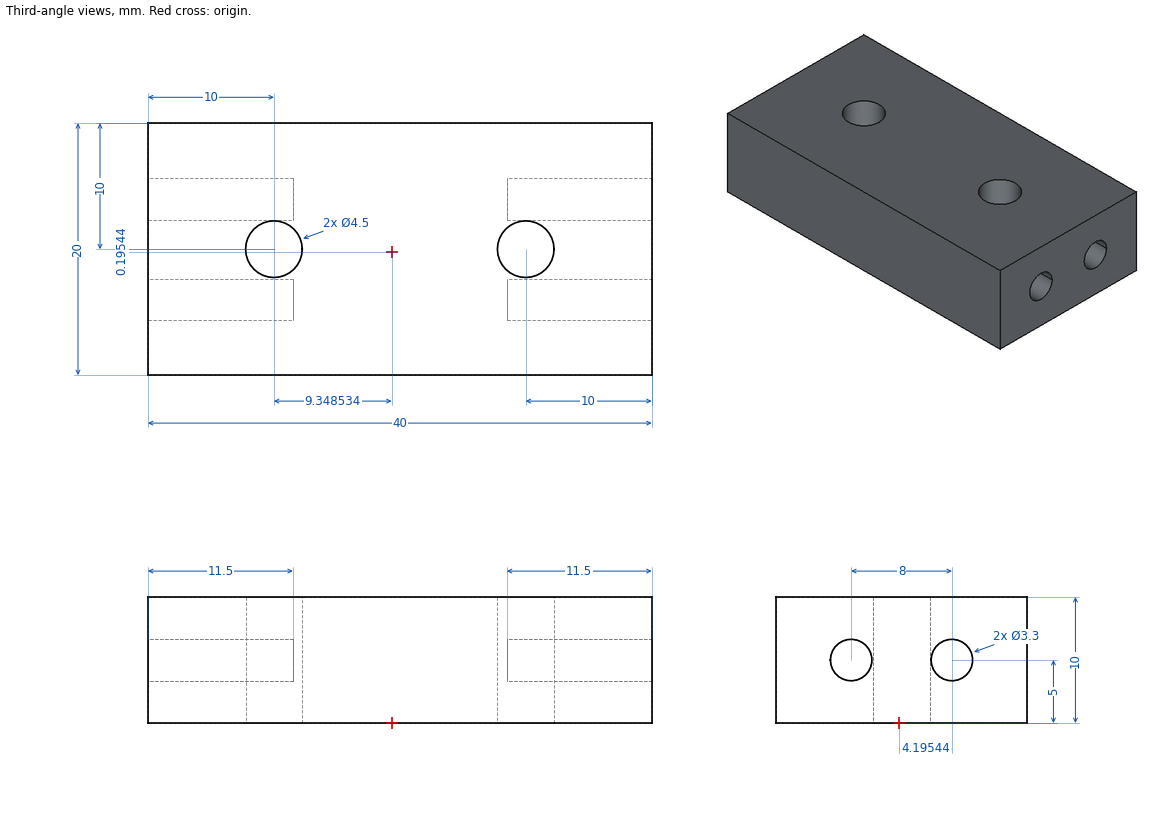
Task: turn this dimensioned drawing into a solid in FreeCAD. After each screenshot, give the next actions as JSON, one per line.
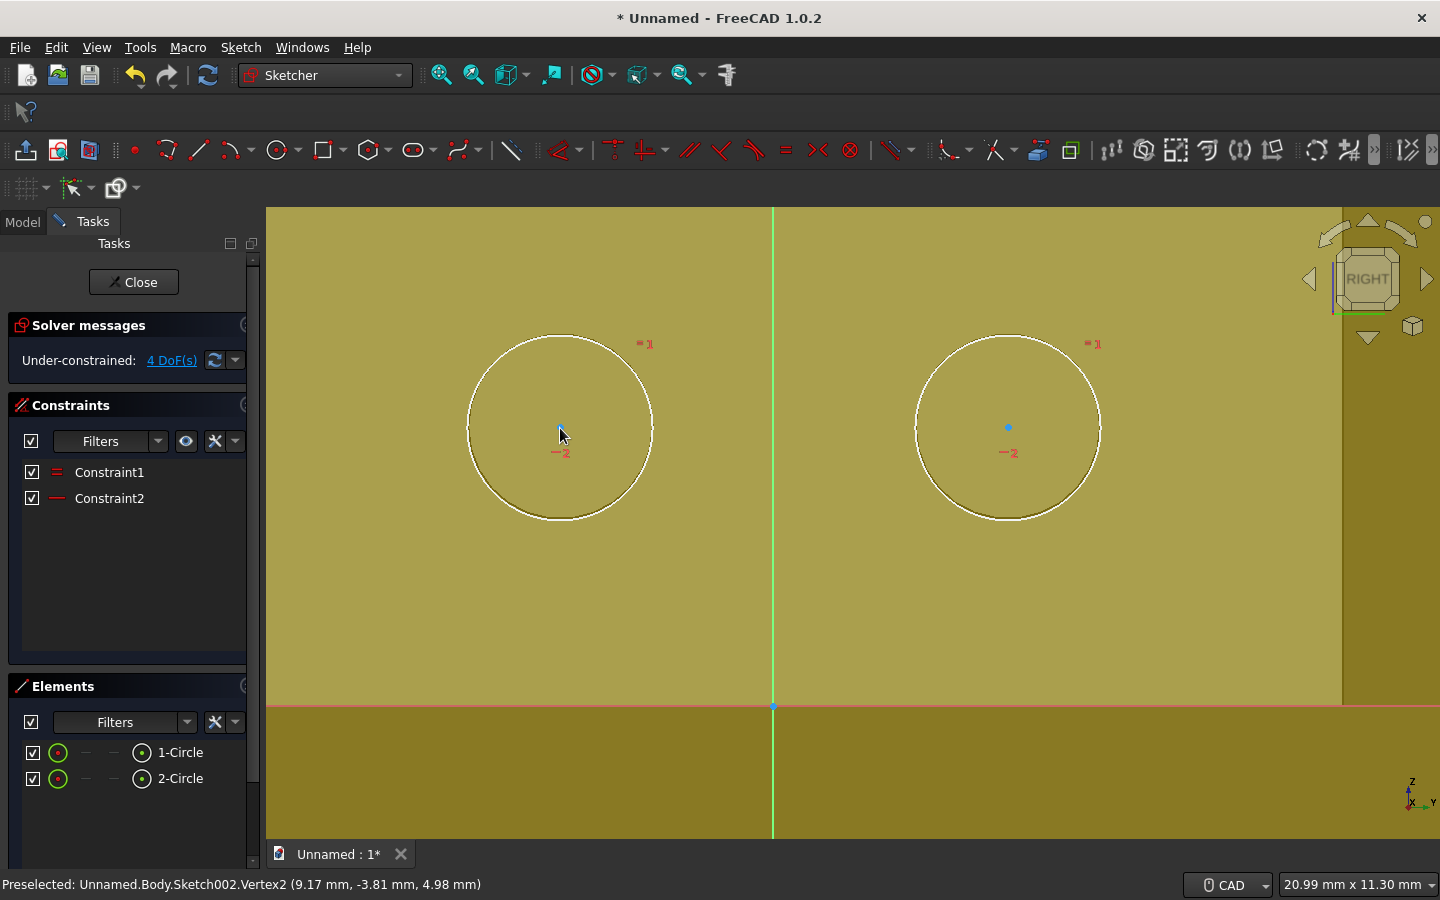
{"action": "key", "text": "d"}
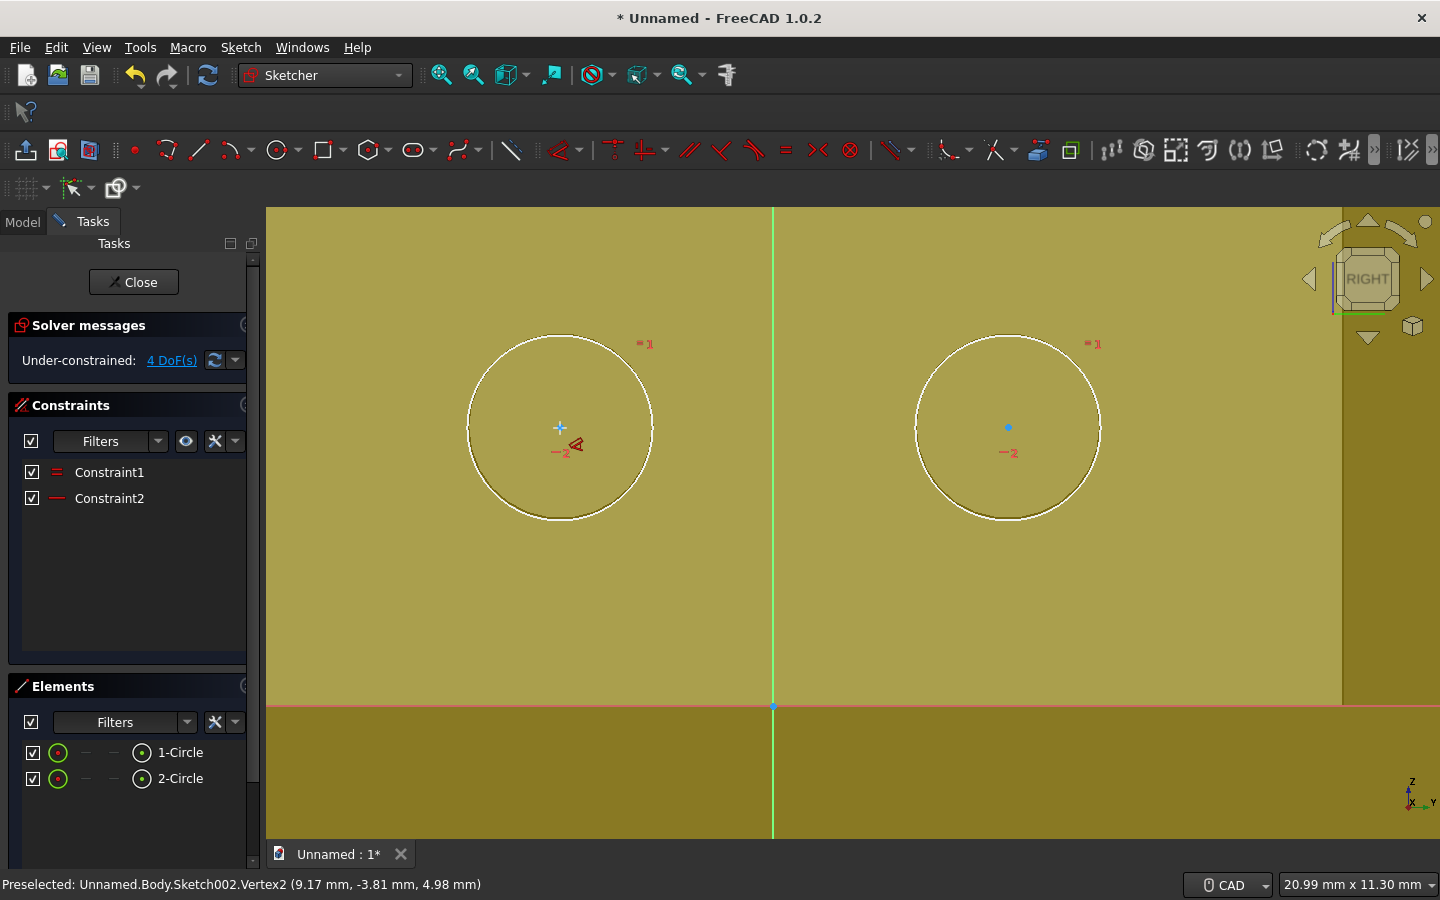
{"action": "left_click", "coordinate": [1073, 362]}
{"action": "left_click", "coordinate": [1095, 339]}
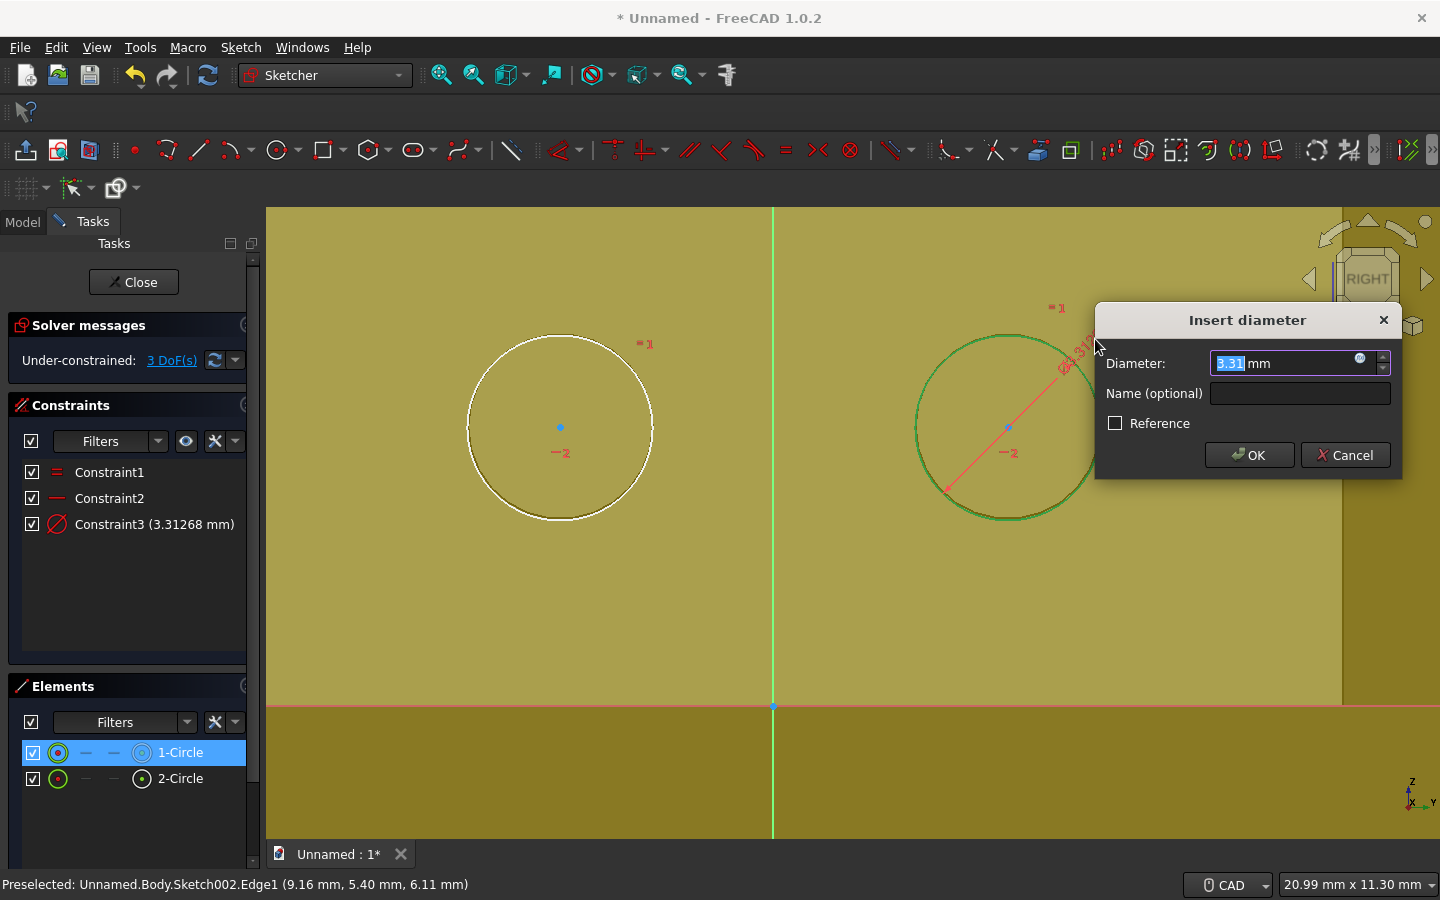
{"action": "type", "text": "3.3"}
{"action": "key", "text": "Return"}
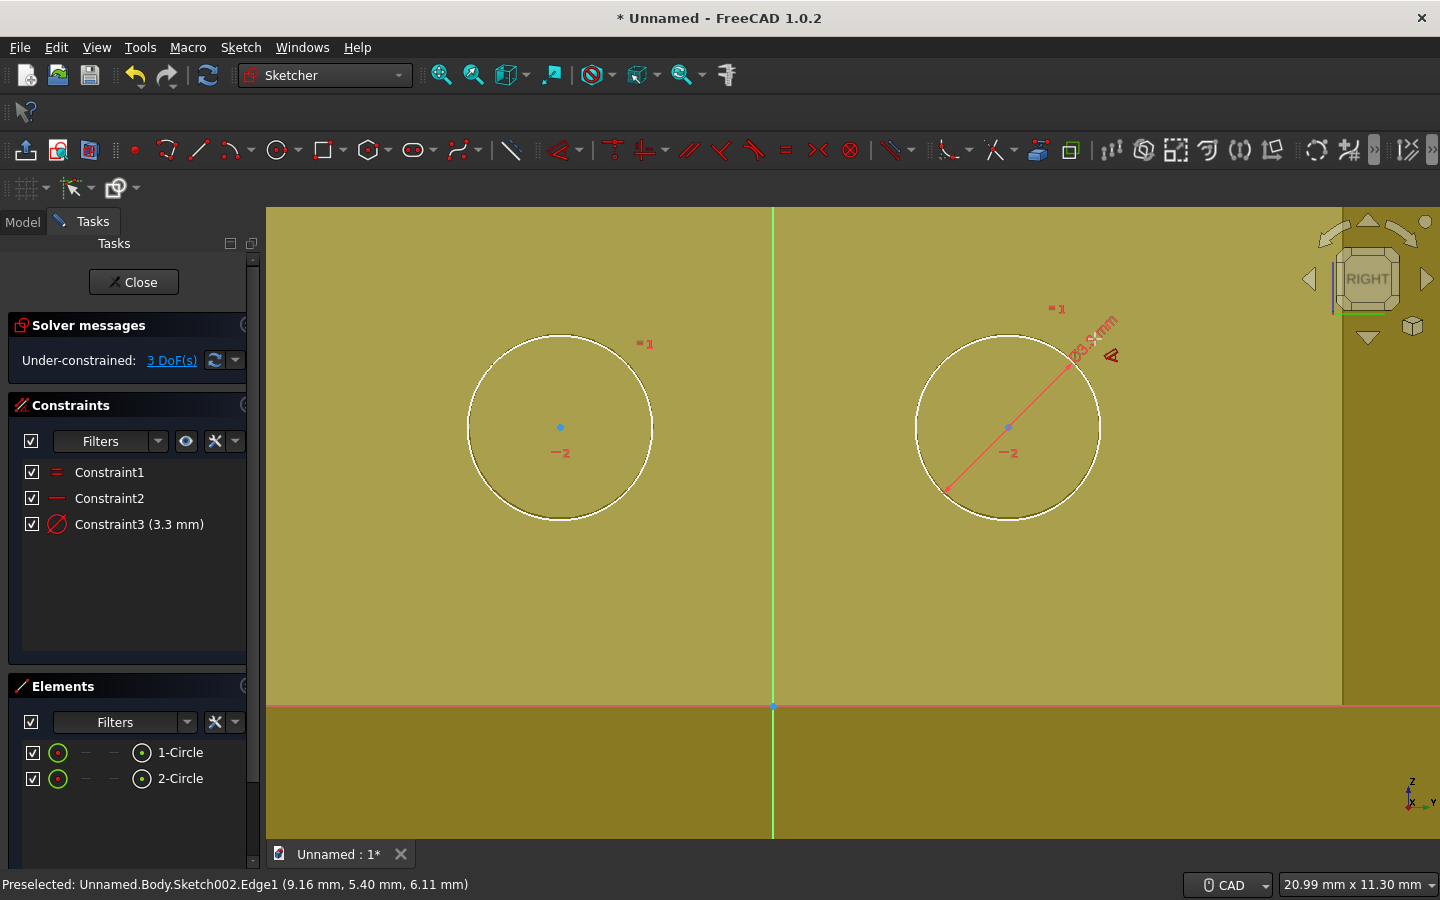
{"action": "left_click", "coordinate": [1008, 428]}
{"action": "left_click", "coordinate": [1042, 567]}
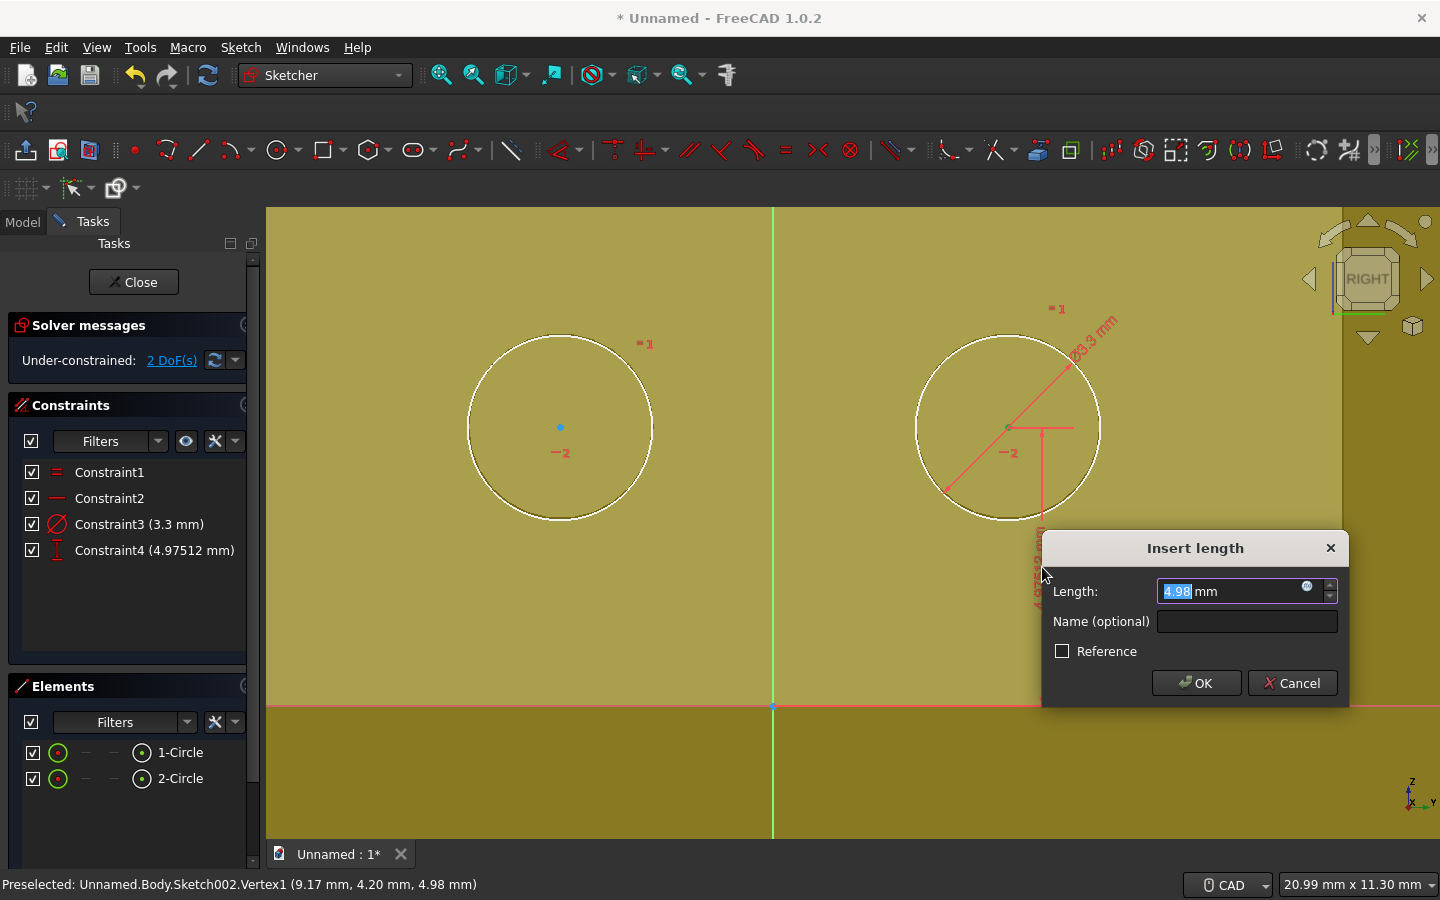
{"action": "type", "text": "5"}
{"action": "key", "text": "Return"}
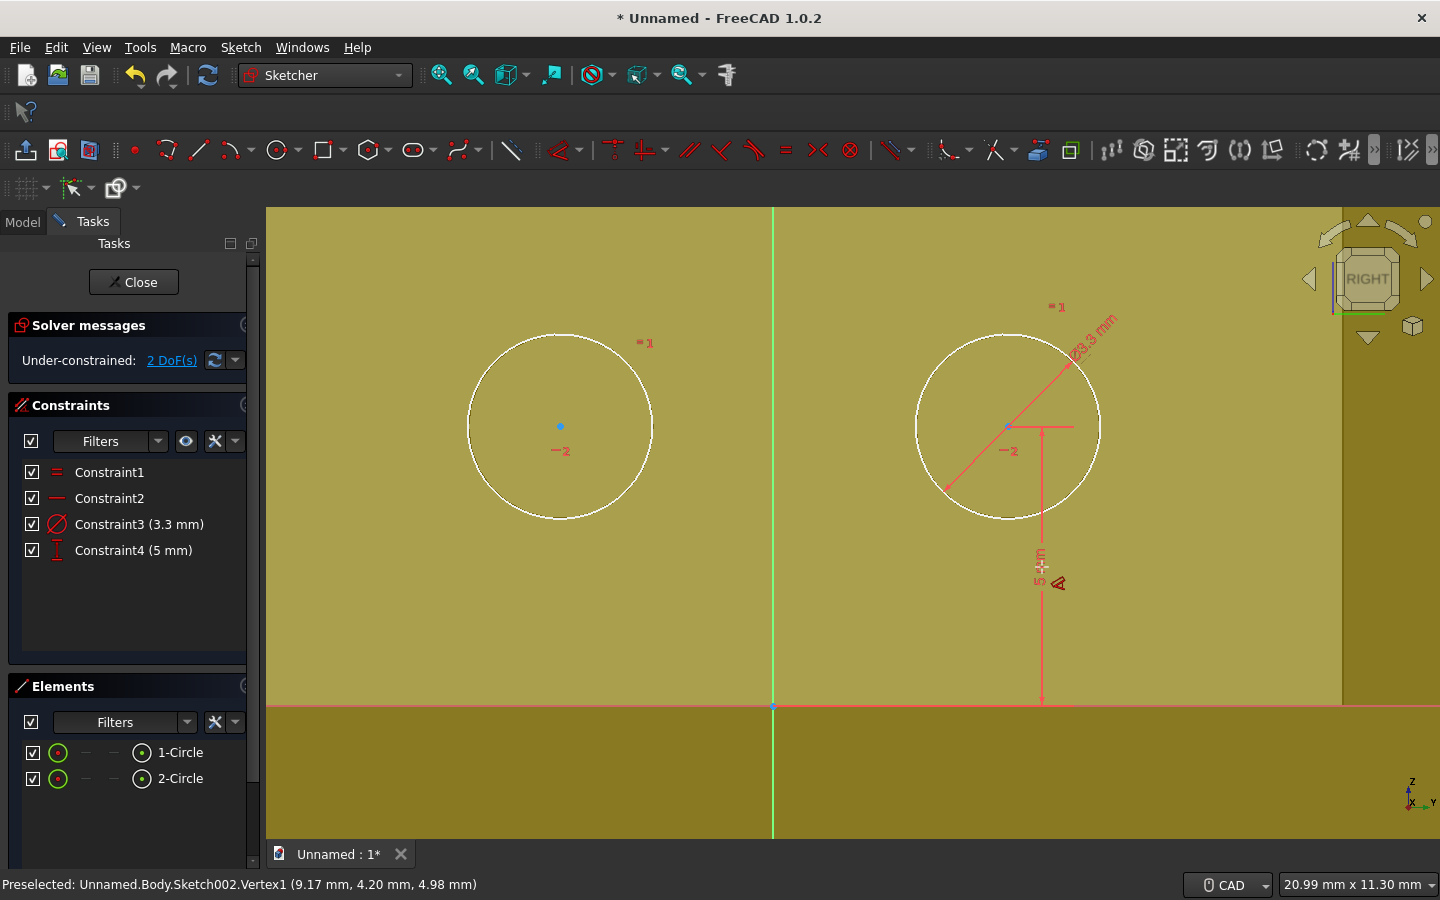
{"action": "left_click", "coordinate": [1008, 427]}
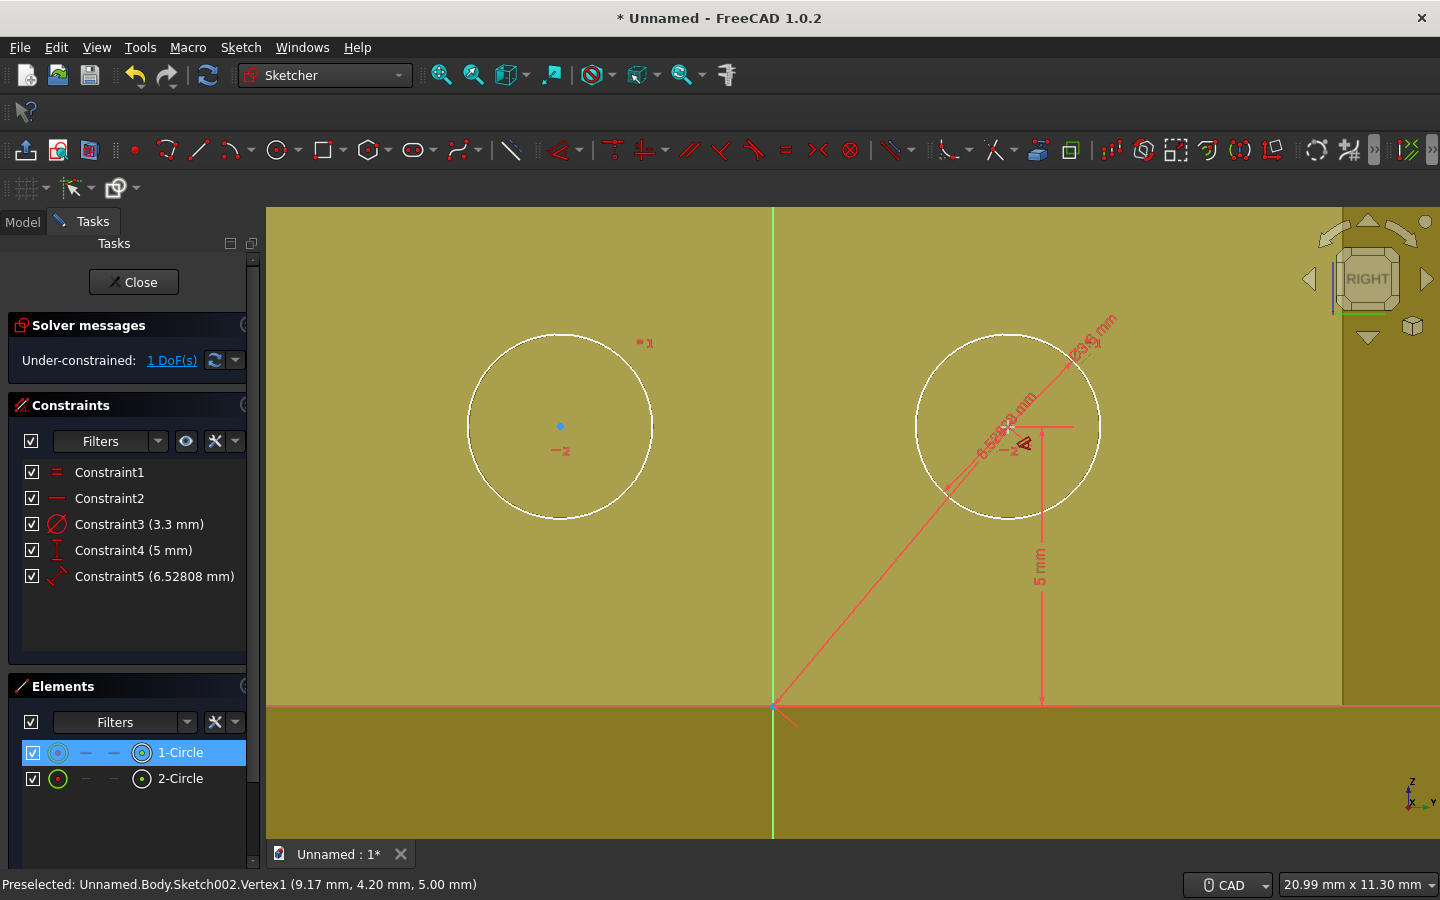
{"action": "left_click", "coordinate": [560, 427]}
{"action": "left_click", "coordinate": [681, 393]}